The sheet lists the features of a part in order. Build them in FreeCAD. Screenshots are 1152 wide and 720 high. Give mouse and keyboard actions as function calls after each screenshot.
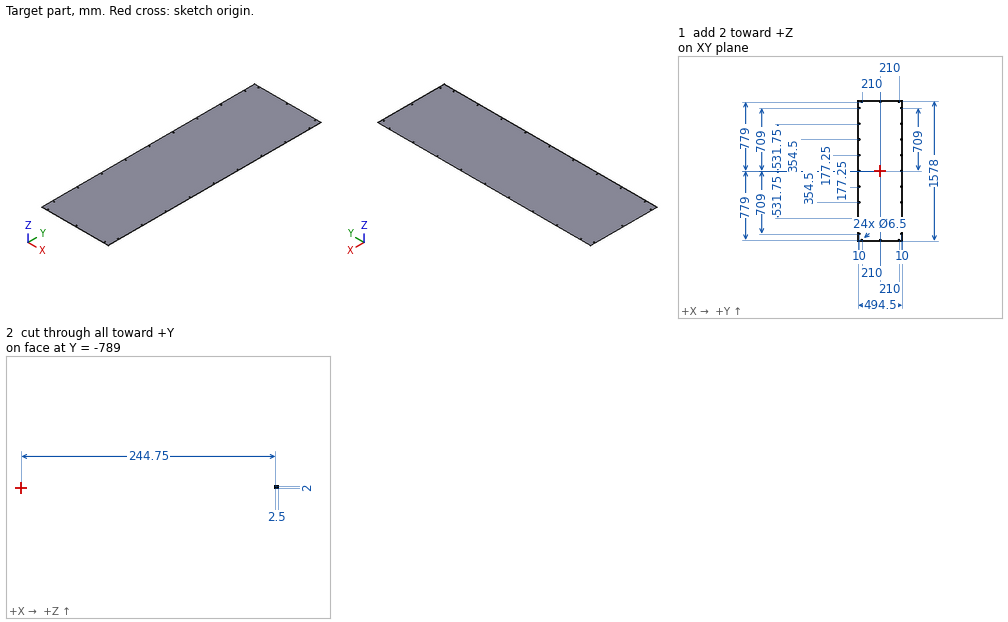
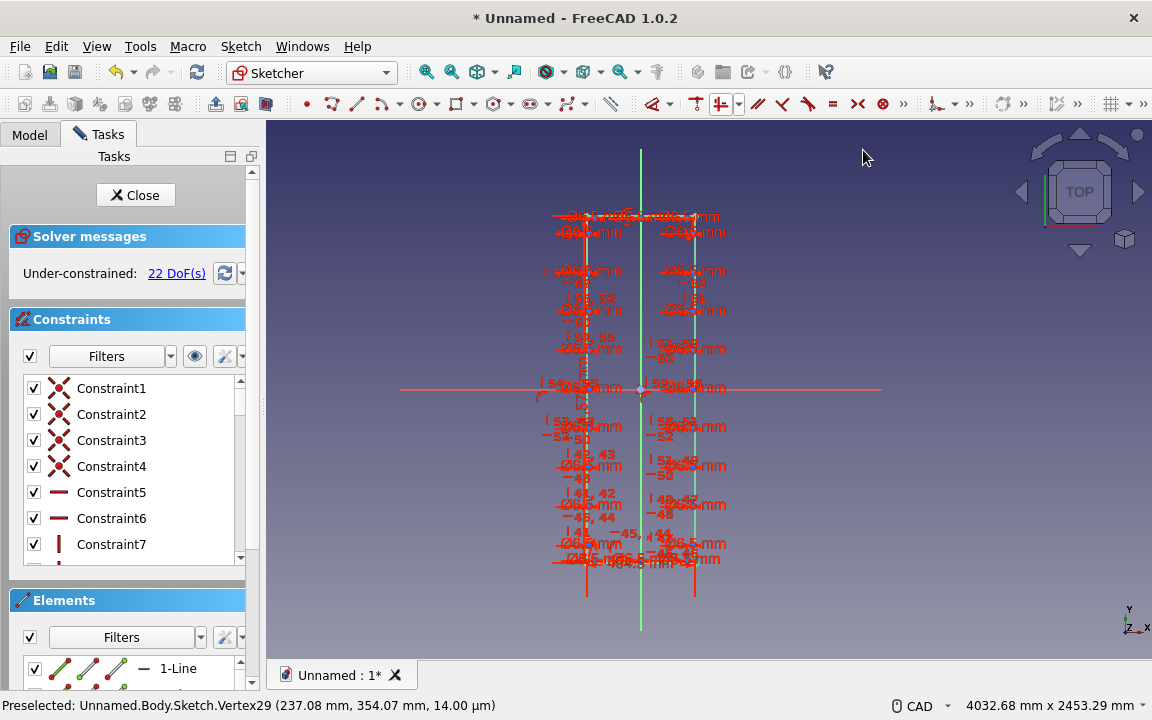
scroll(595, 219, up, 2)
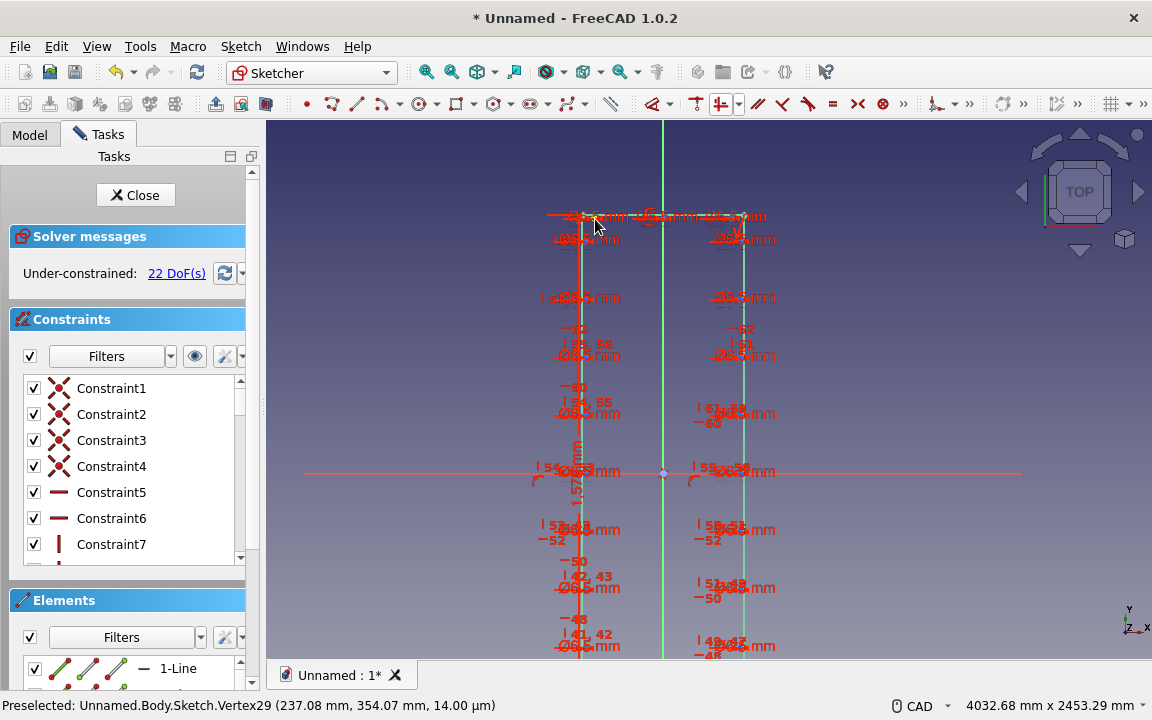
click(594, 219)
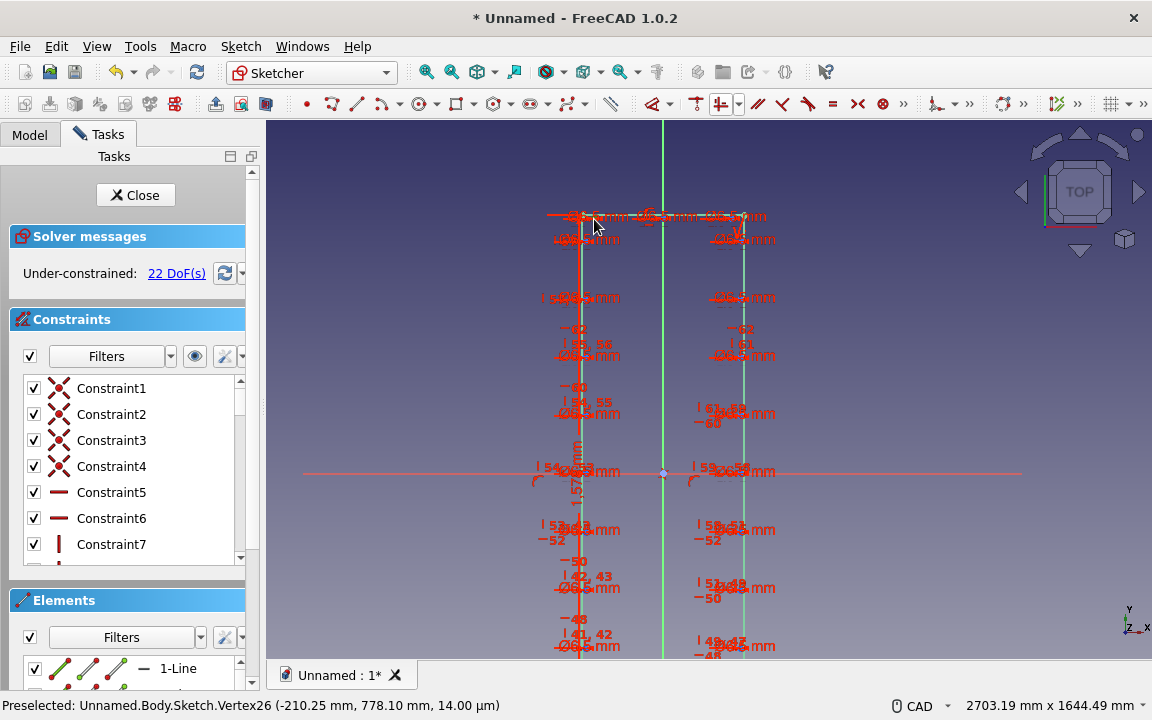
click(663, 219)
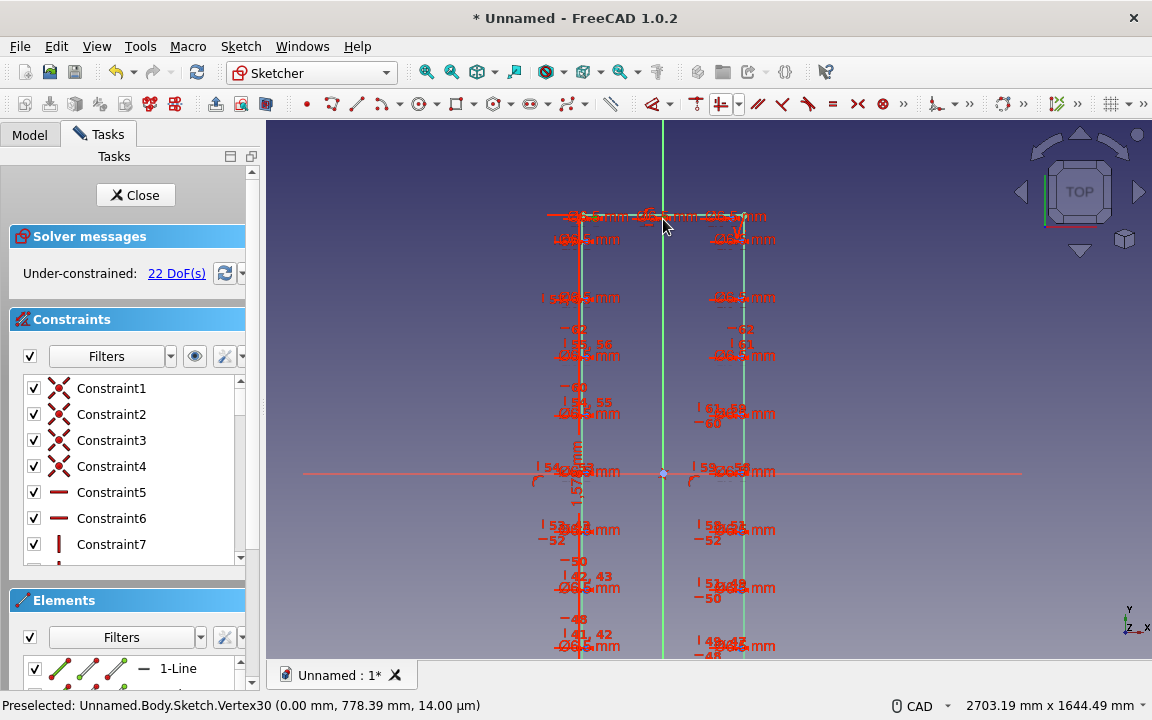
click(738, 104)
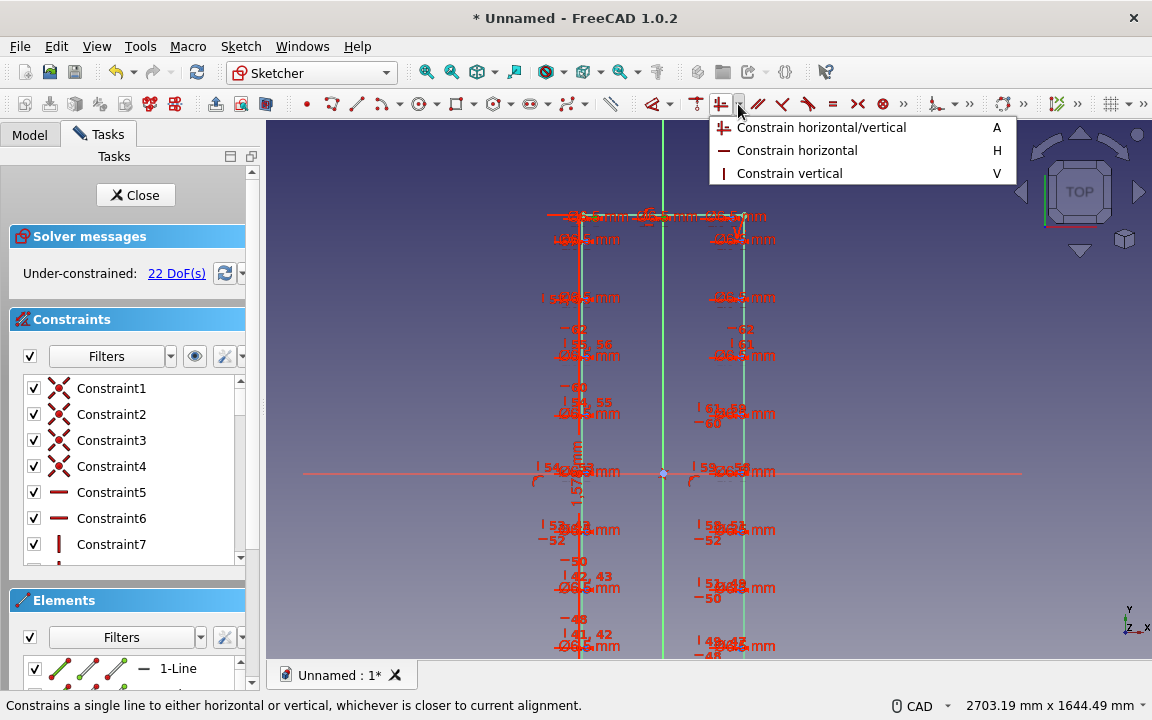
click(863, 150)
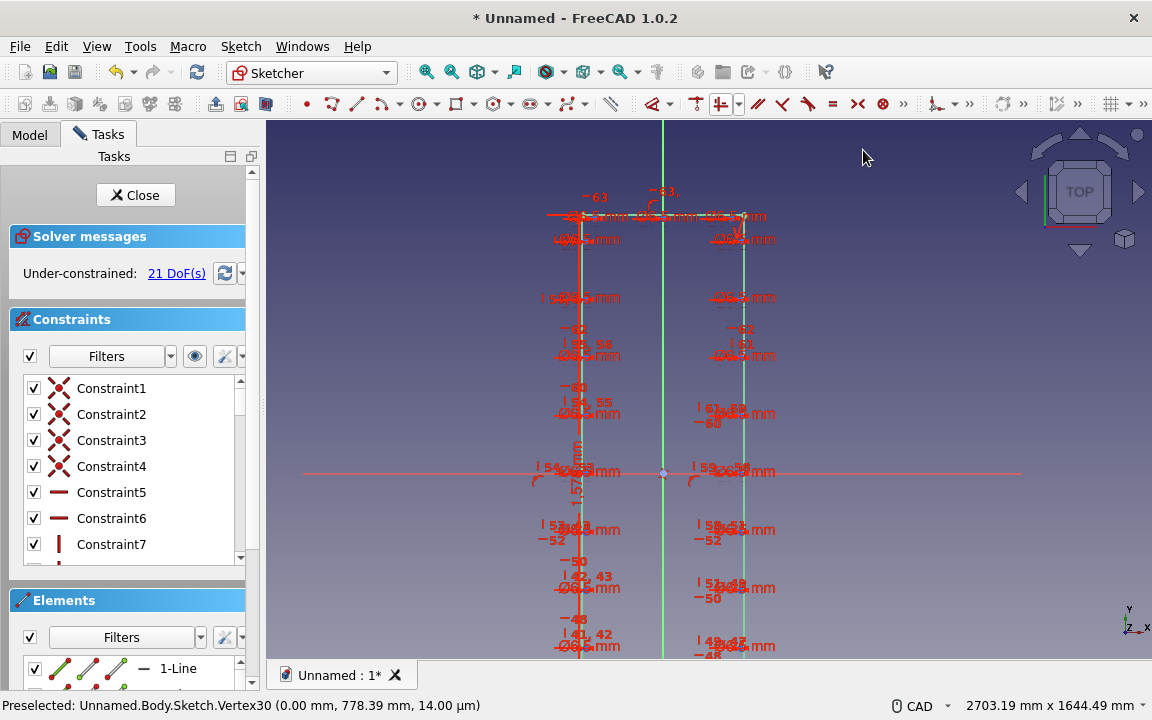
click(741, 358)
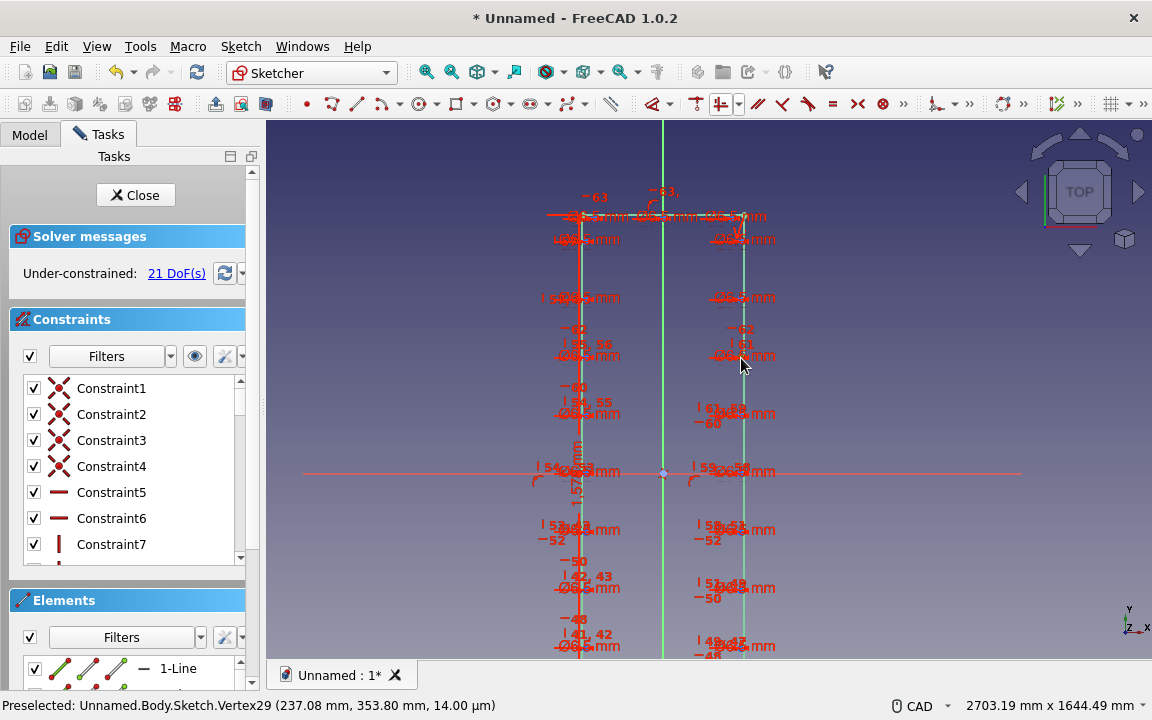
click(741, 300)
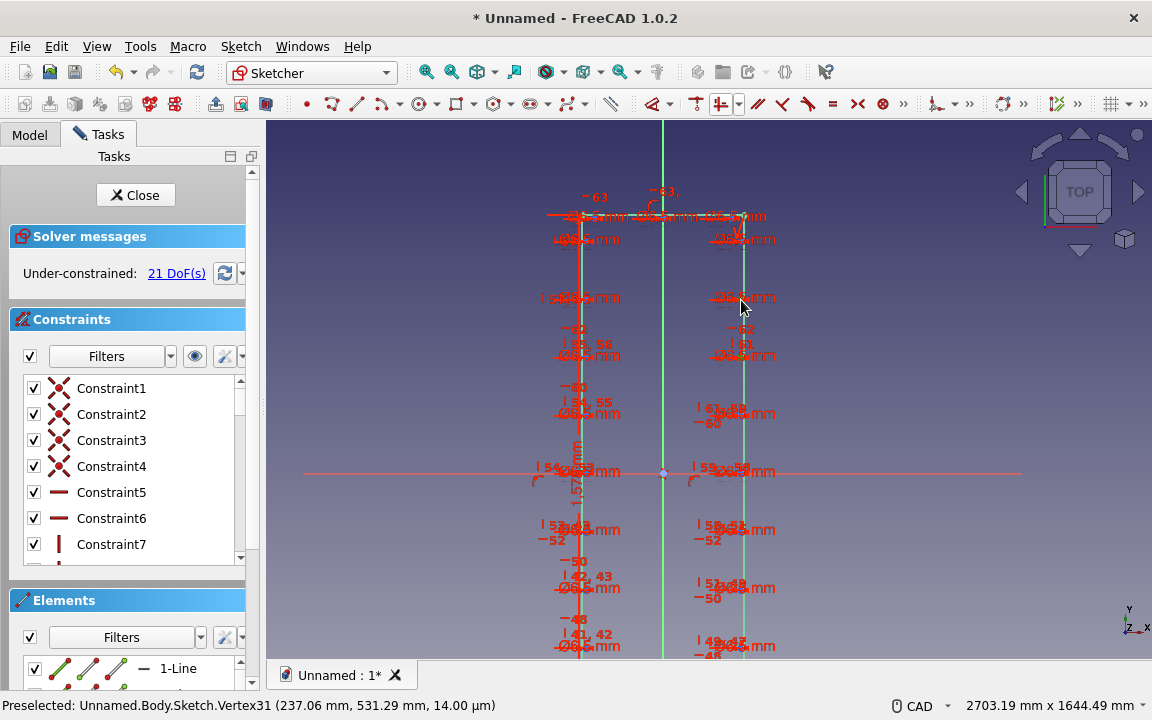
key(v)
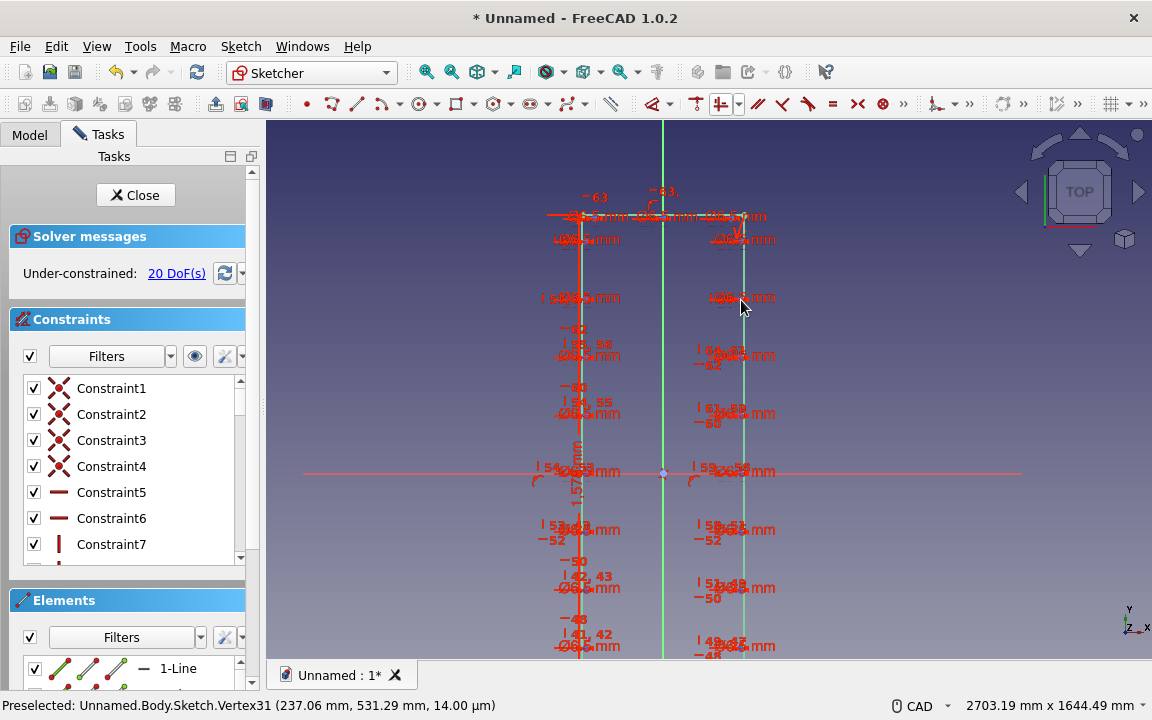
click(586, 300)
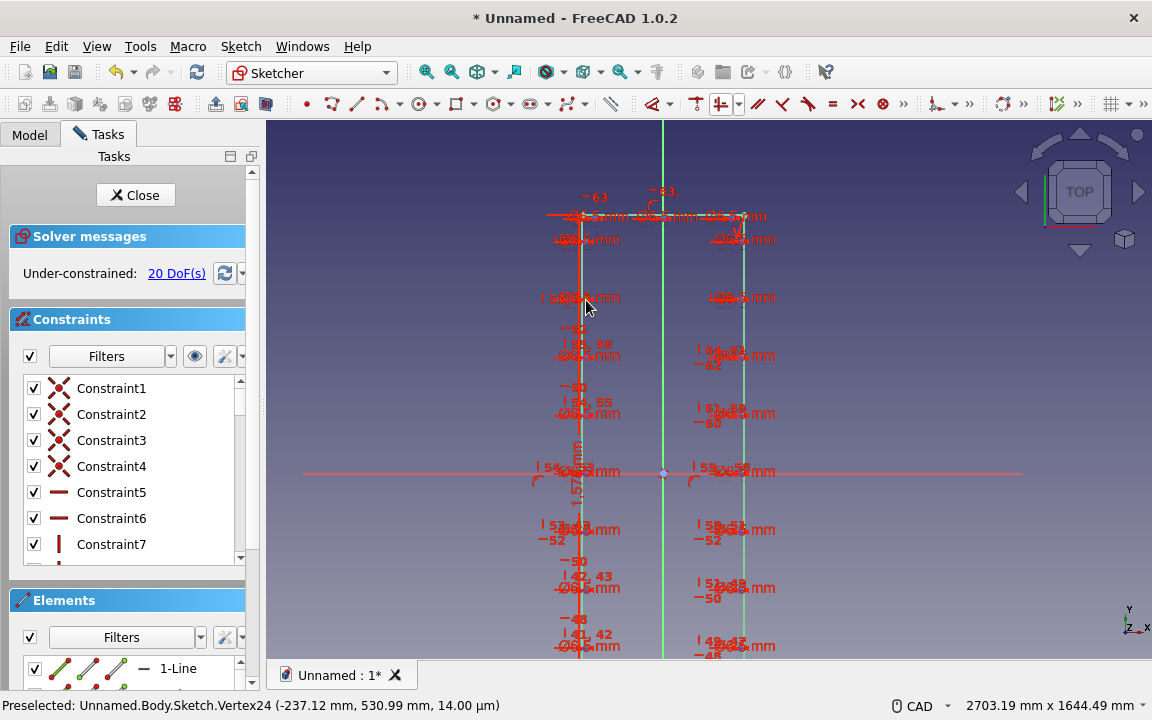
click(741, 300)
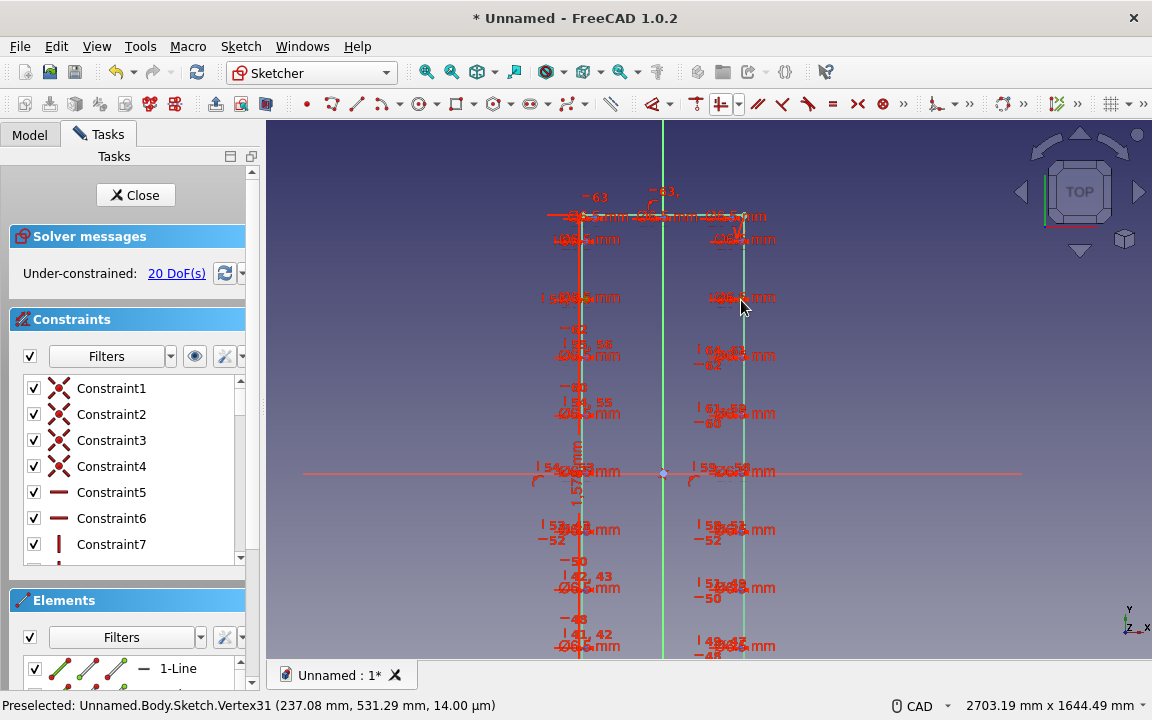
click(738, 104)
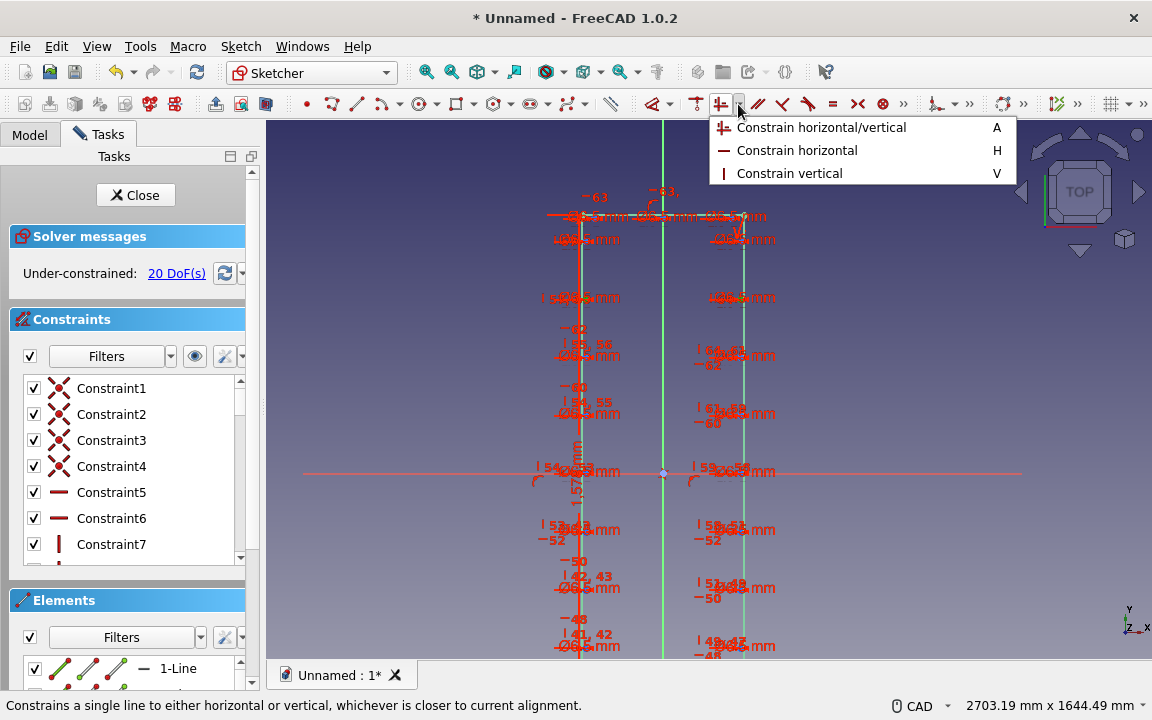
click(863, 150)